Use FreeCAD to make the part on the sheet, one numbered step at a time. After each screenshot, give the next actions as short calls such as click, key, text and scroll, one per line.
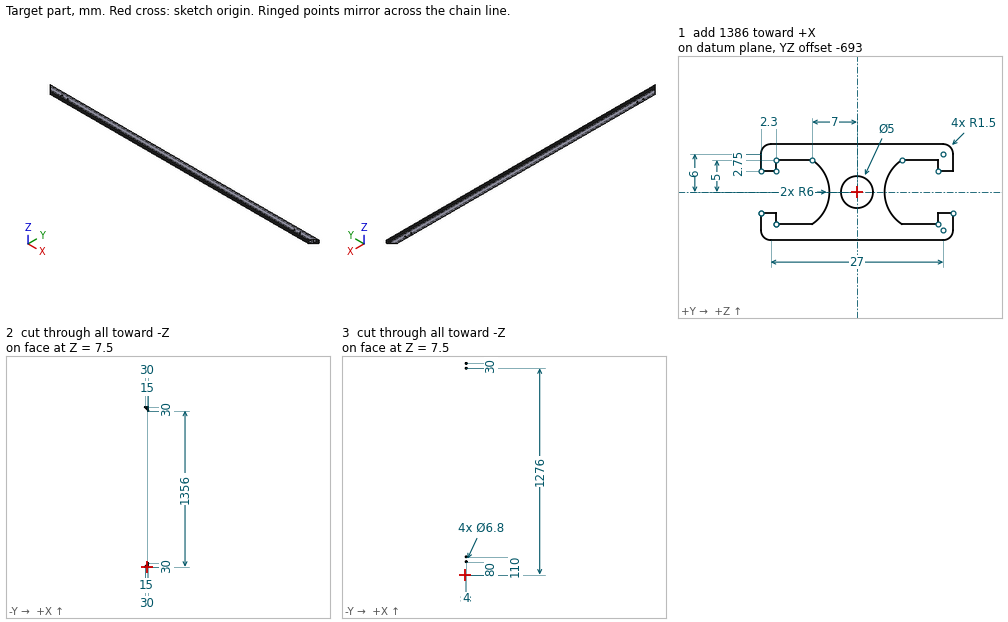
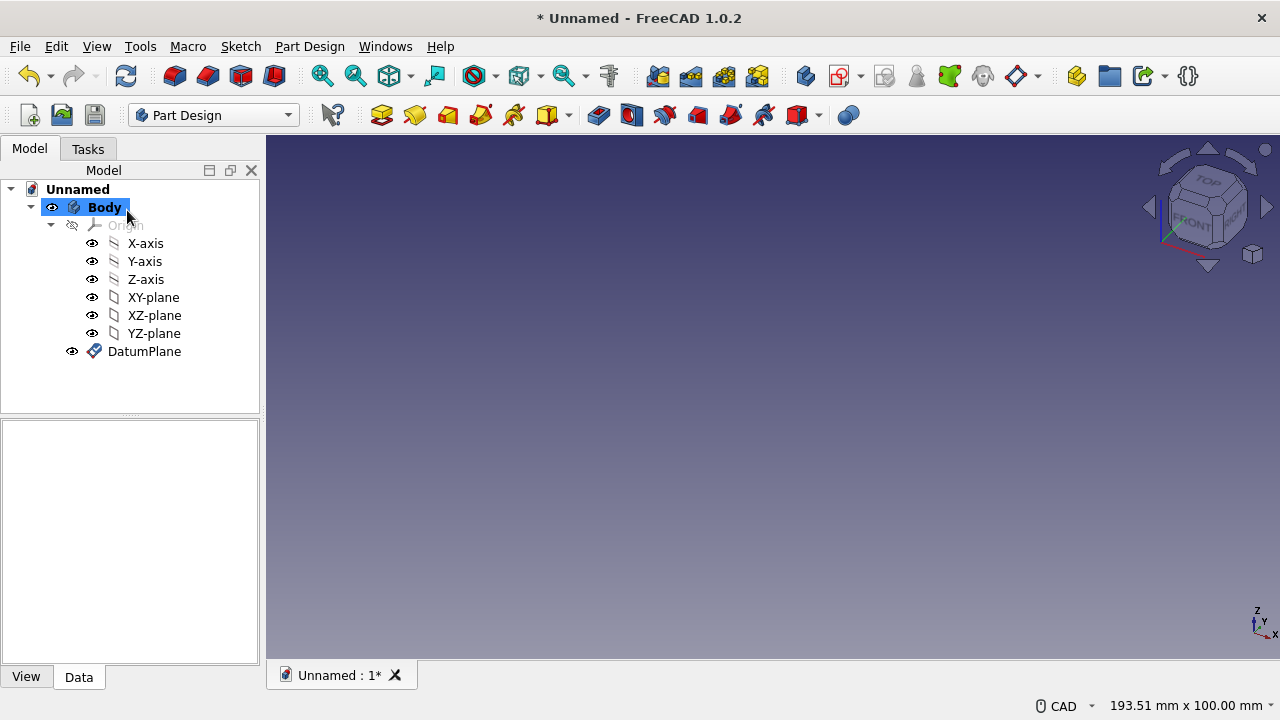
click(117, 351)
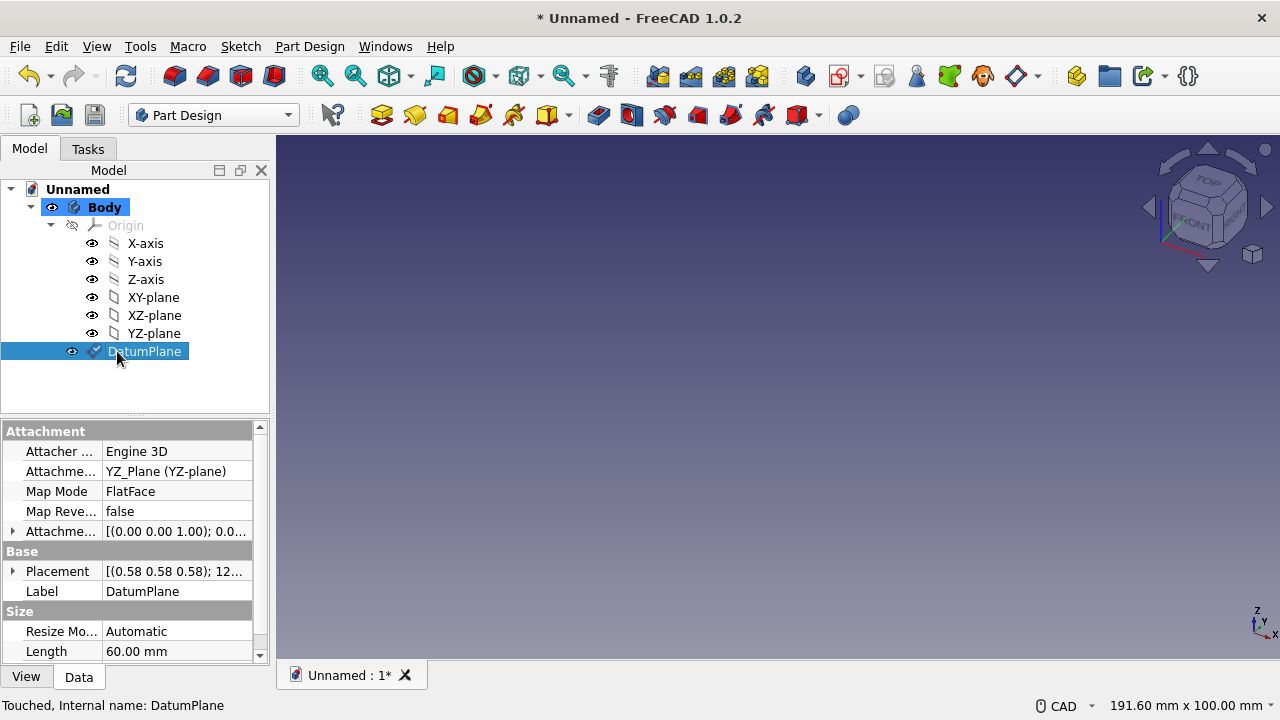
click(838, 76)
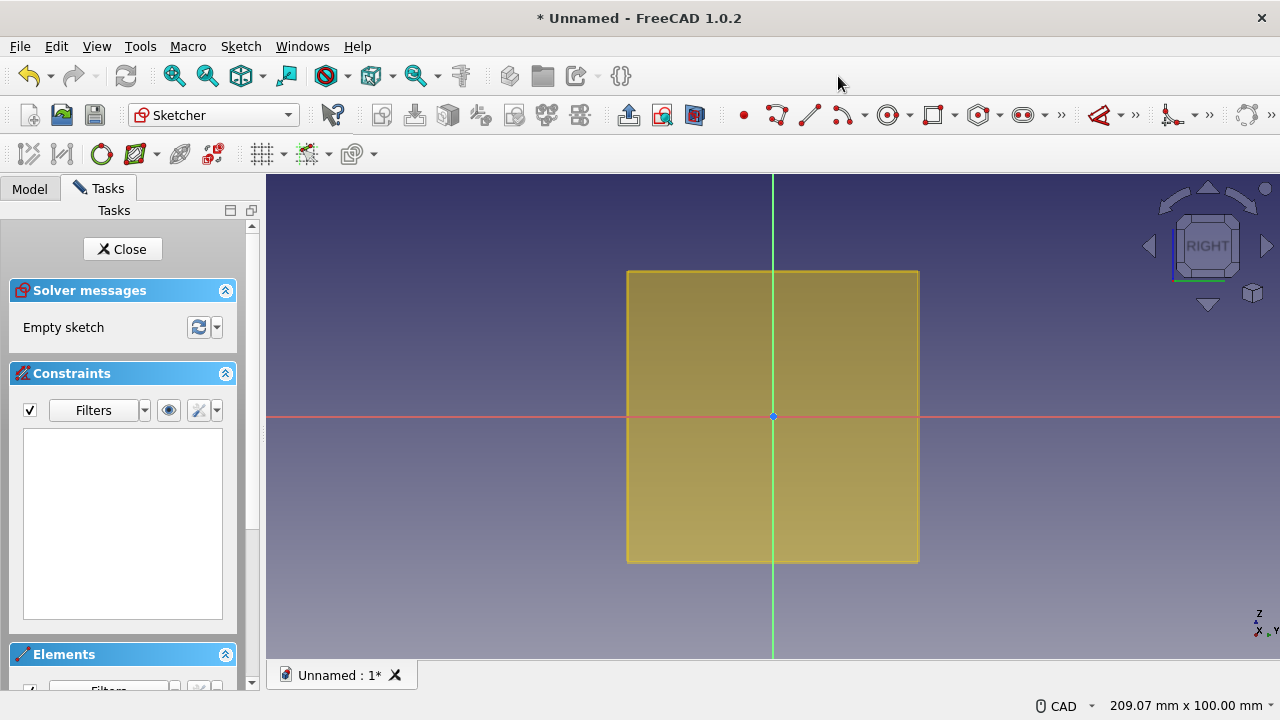
scroll(795, 416, up, 7)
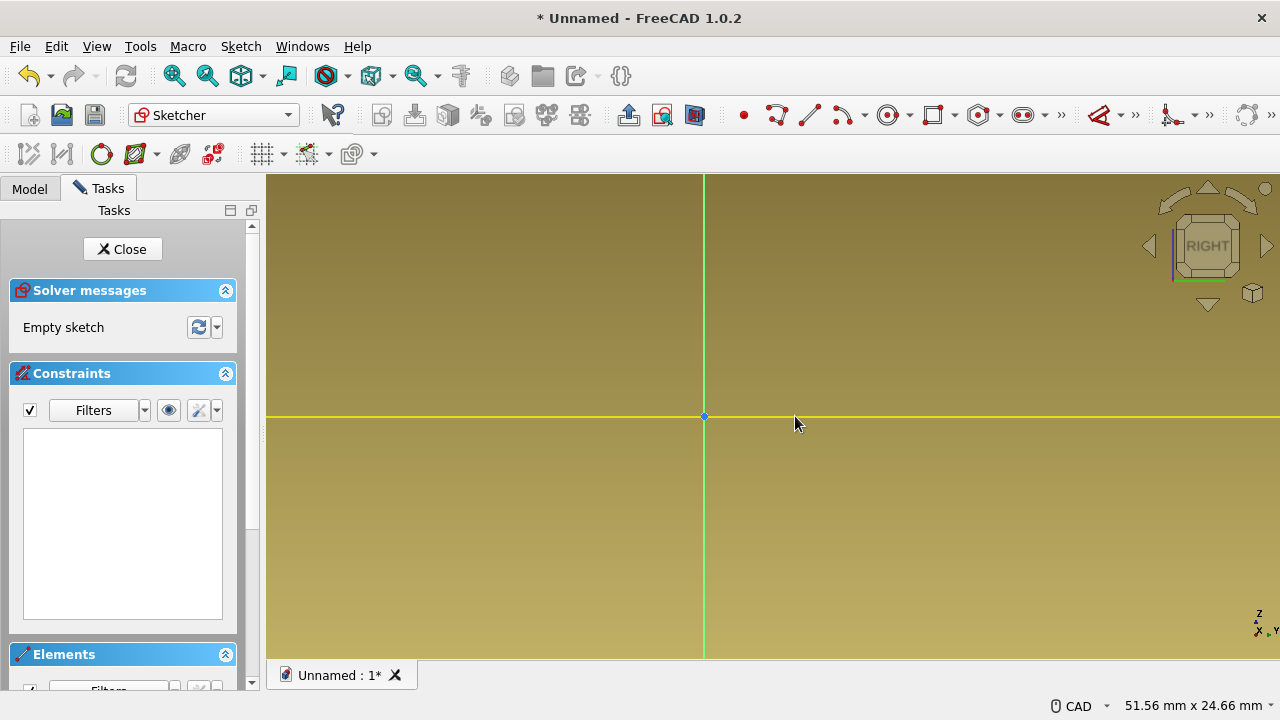
click(777, 116)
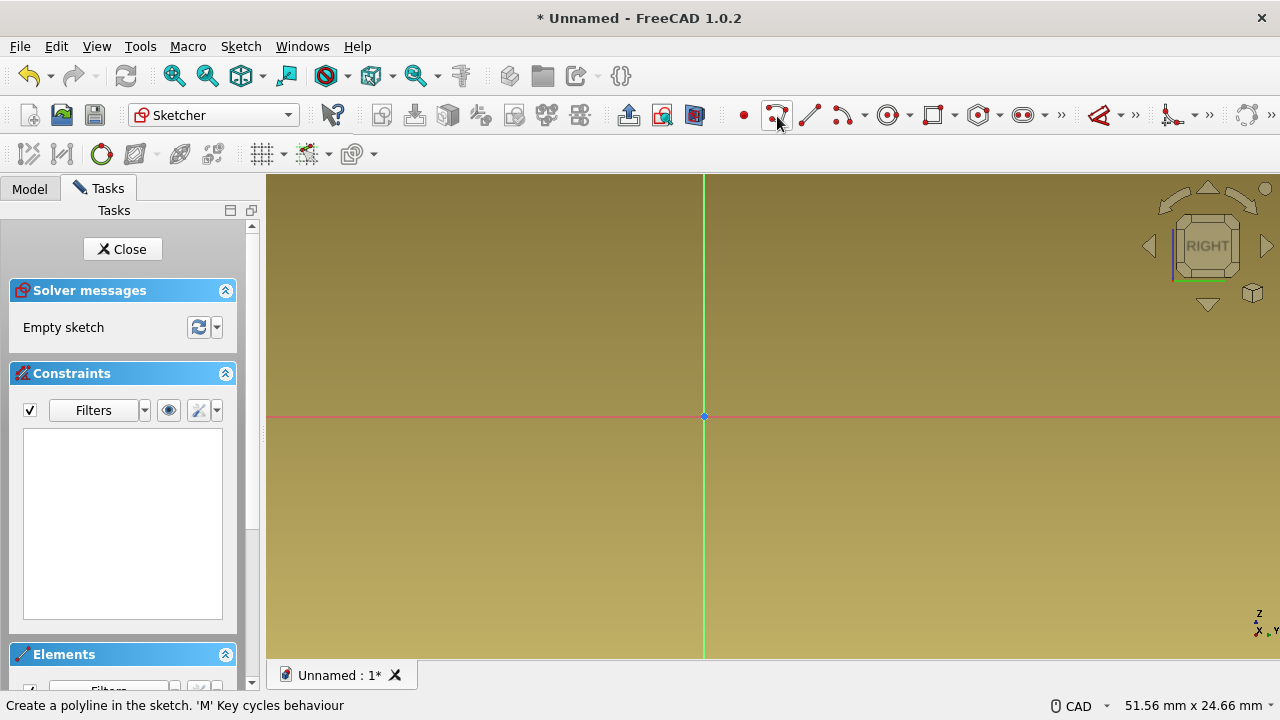
click(409, 298)
click(409, 353)
click(454, 353)
click(454, 318)
click(567, 318)
right_click(567, 318)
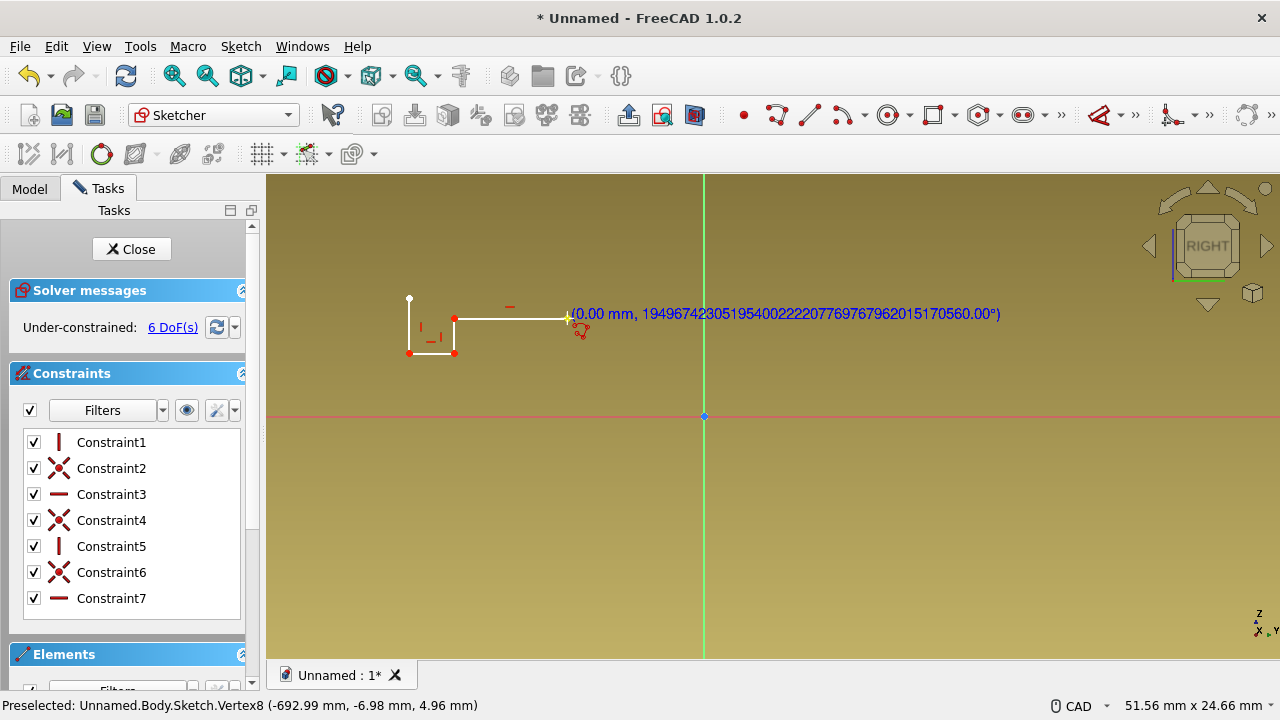
click(567, 515)
click(454, 515)
click(454, 480)
click(409, 480)
click(409, 535)
right_click(409, 535)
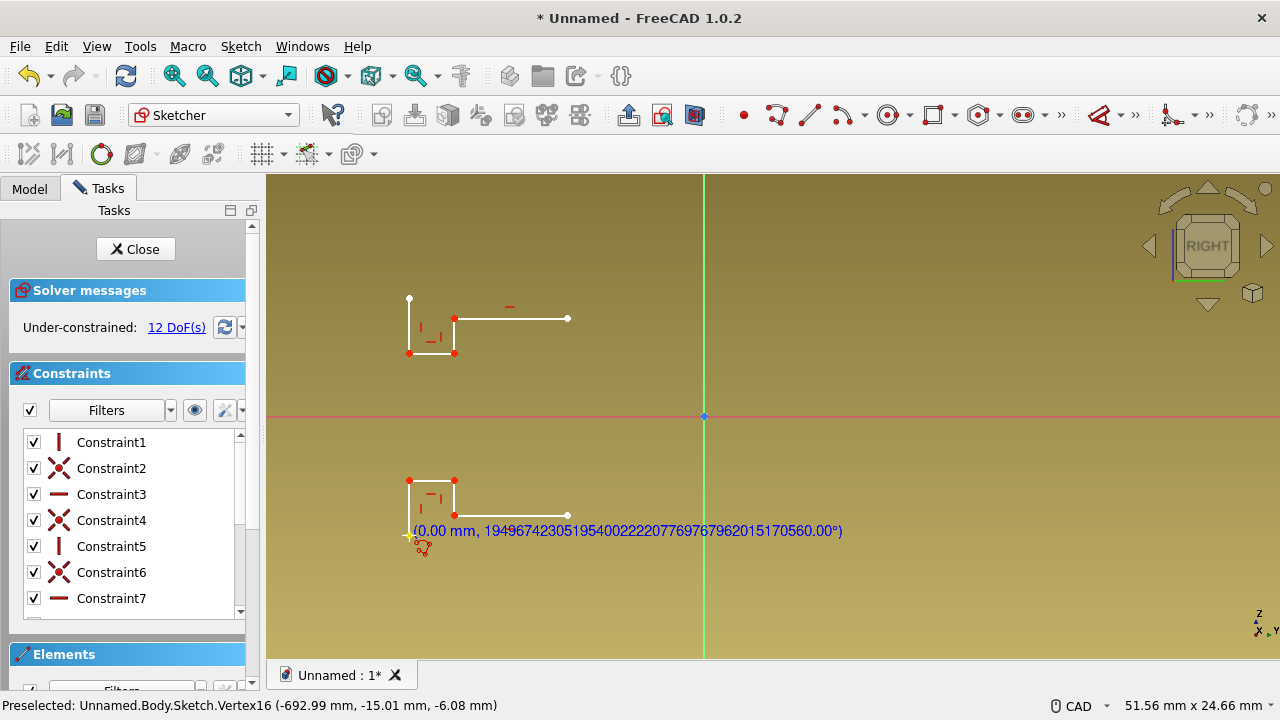
click(810, 116)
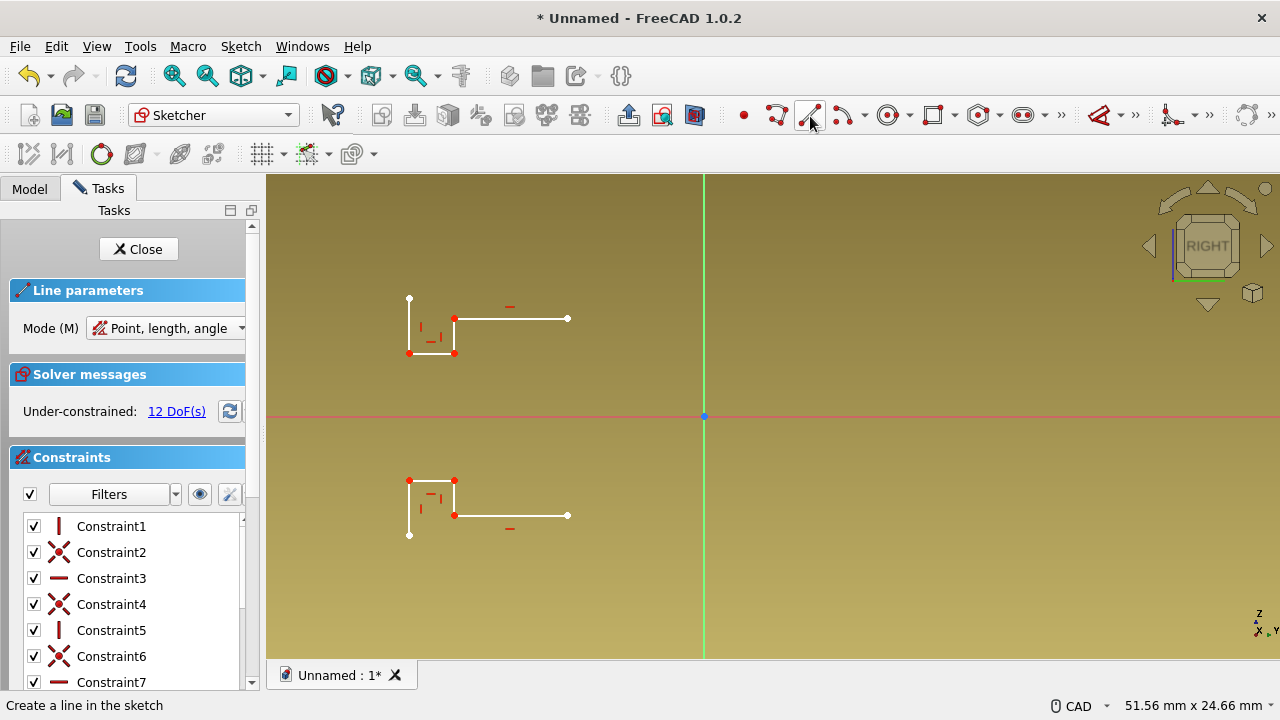
click(439, 564)
click(970, 564)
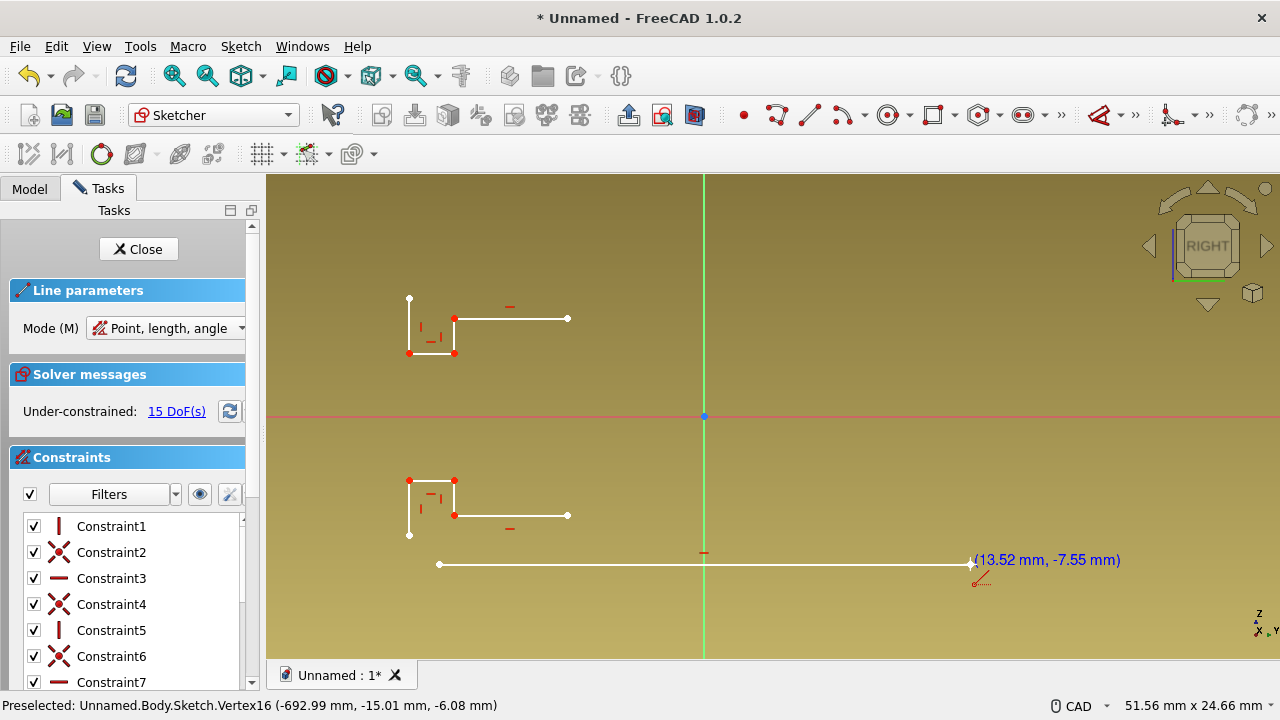
key(g)
key(m)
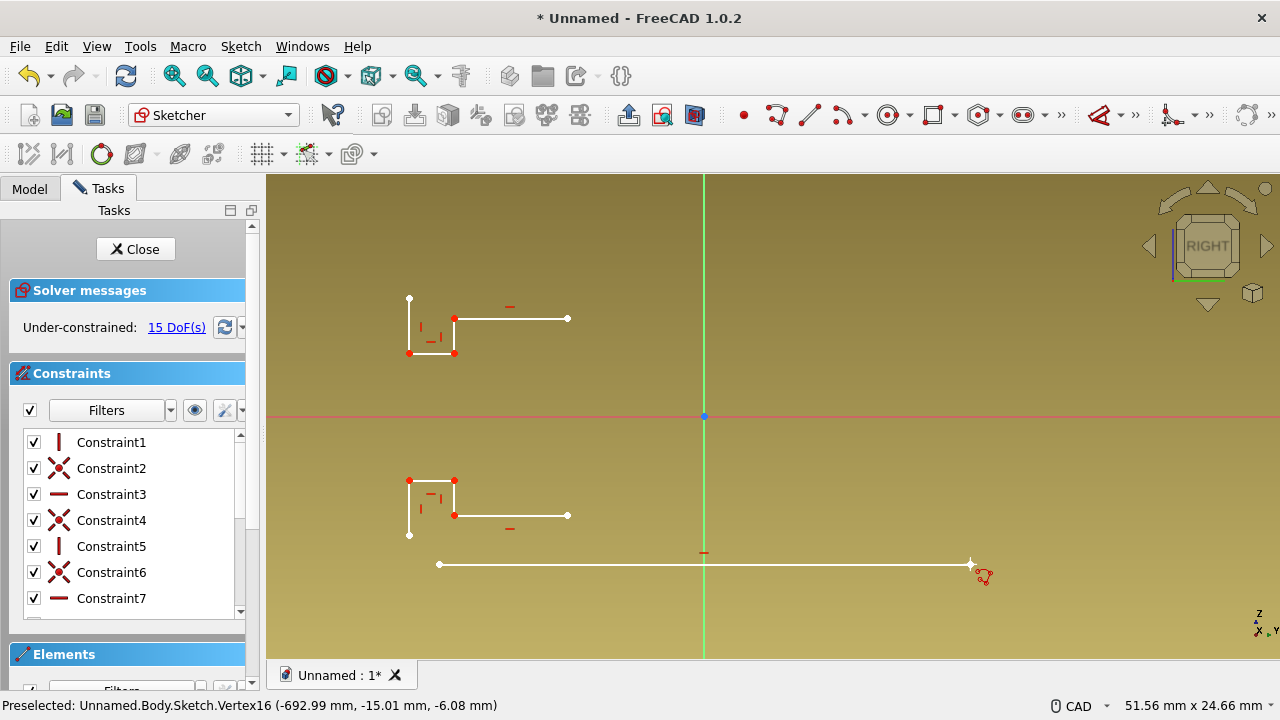
click(999, 535)
click(999, 480)
click(954, 480)
click(954, 515)
click(842, 515)
right_click(842, 515)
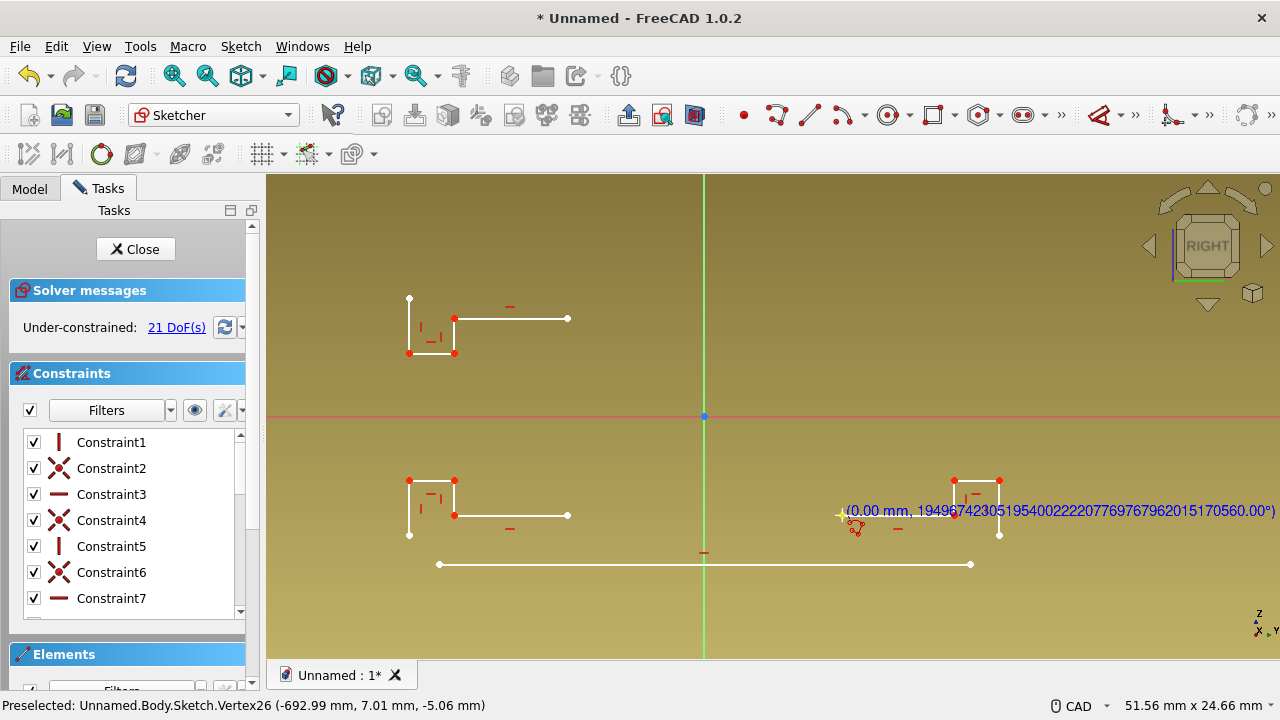
click(842, 318)
click(954, 318)
click(954, 353)
click(999, 353)
click(999, 298)
right_click(999, 298)